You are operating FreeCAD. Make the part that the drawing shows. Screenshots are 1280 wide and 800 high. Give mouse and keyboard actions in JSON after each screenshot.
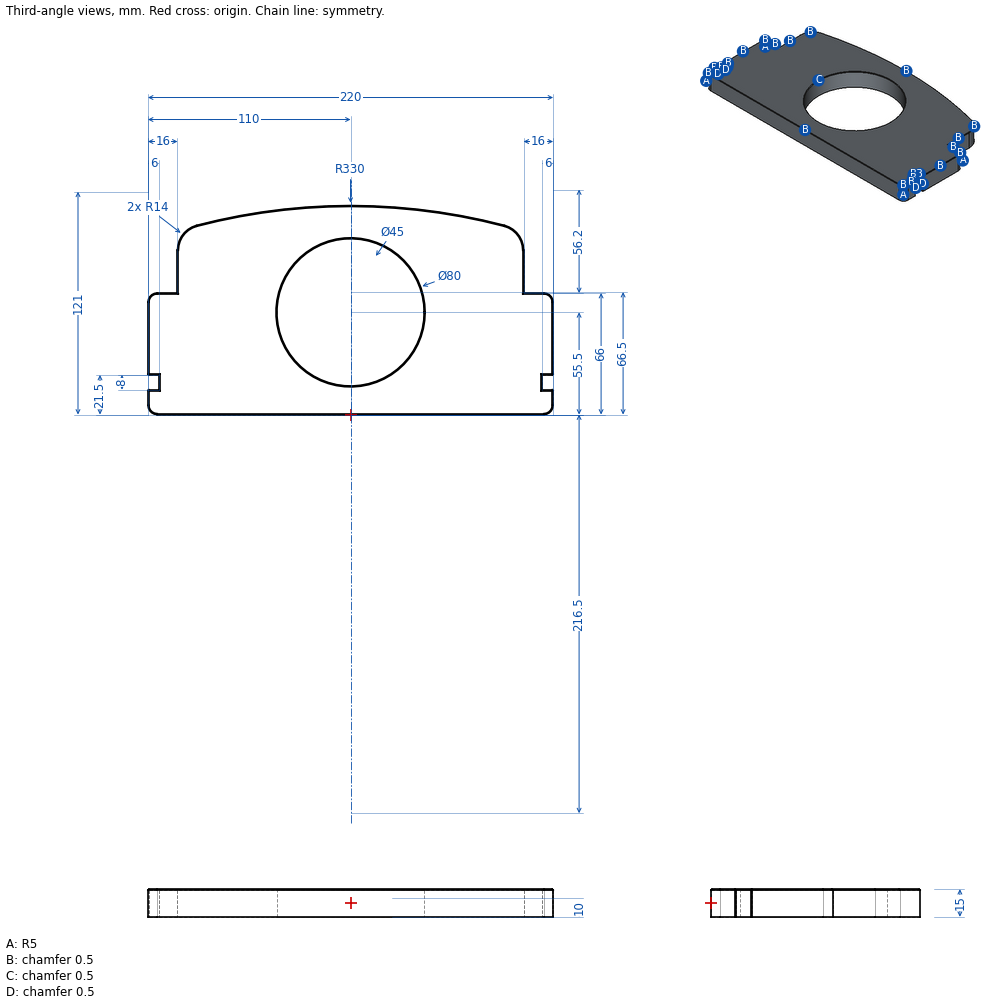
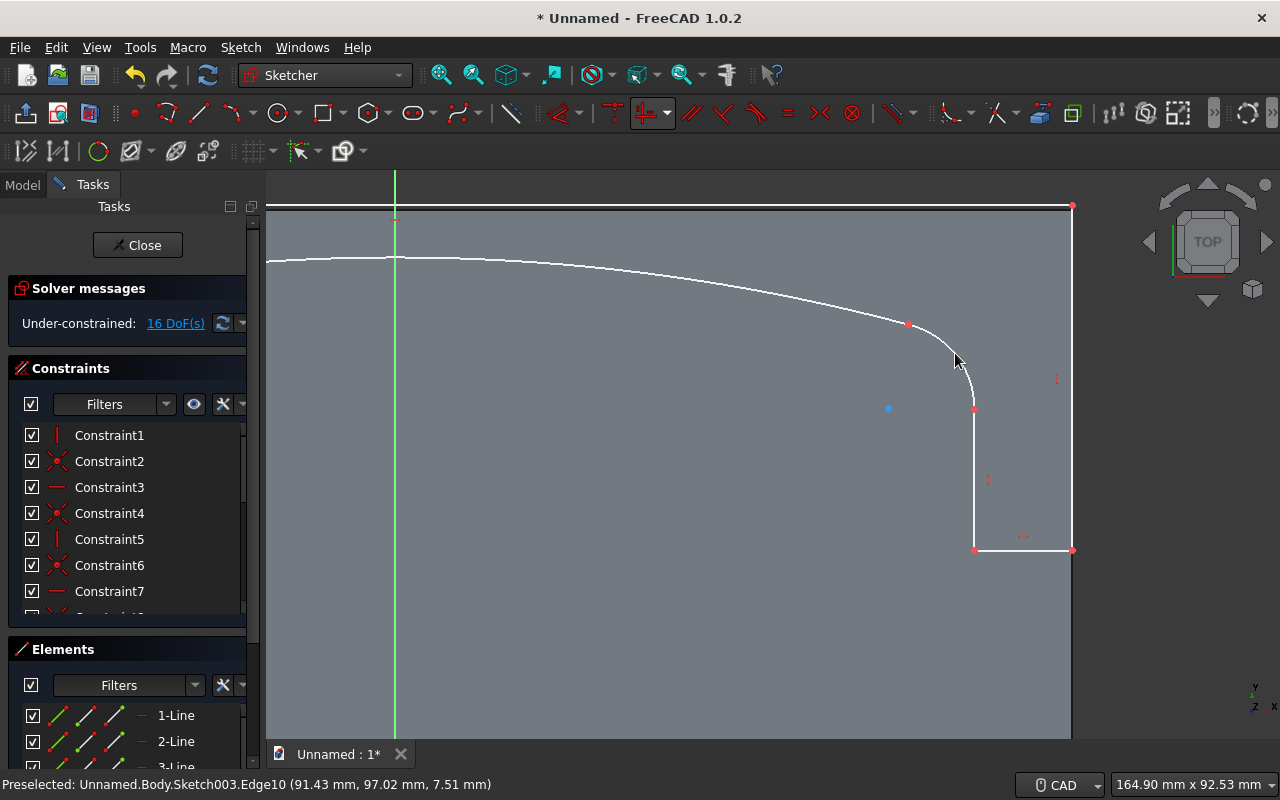
{"action": "left_click", "coordinate": [974, 452]}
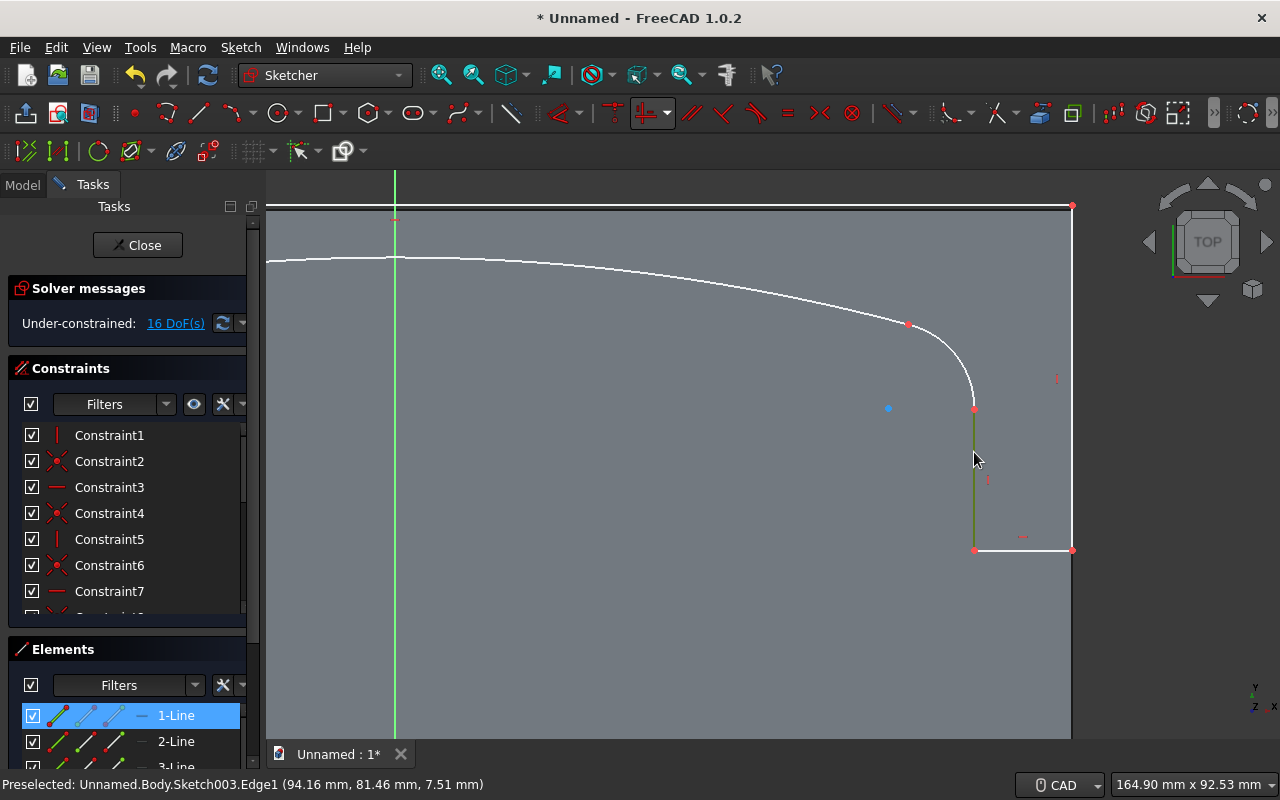
{"action": "left_click", "coordinate": [968, 375]}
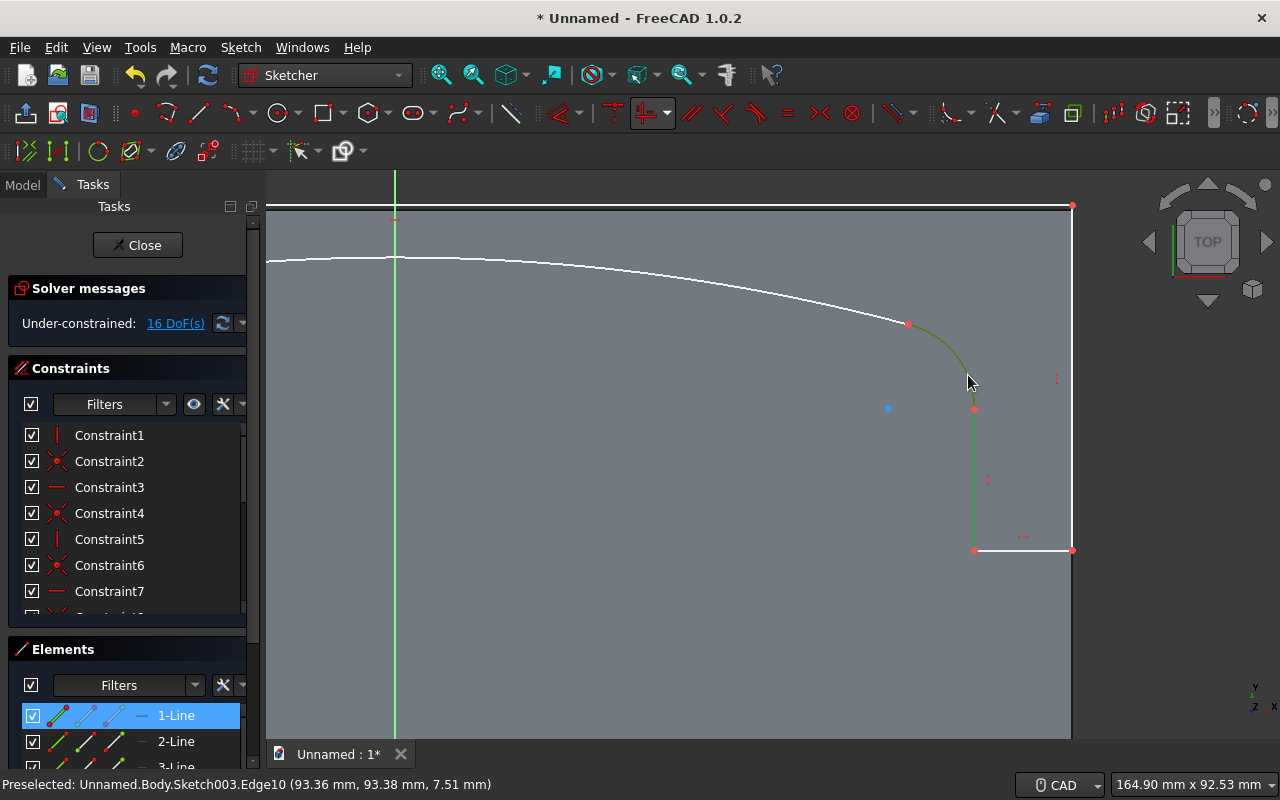
{"action": "left_click", "coordinate": [756, 114]}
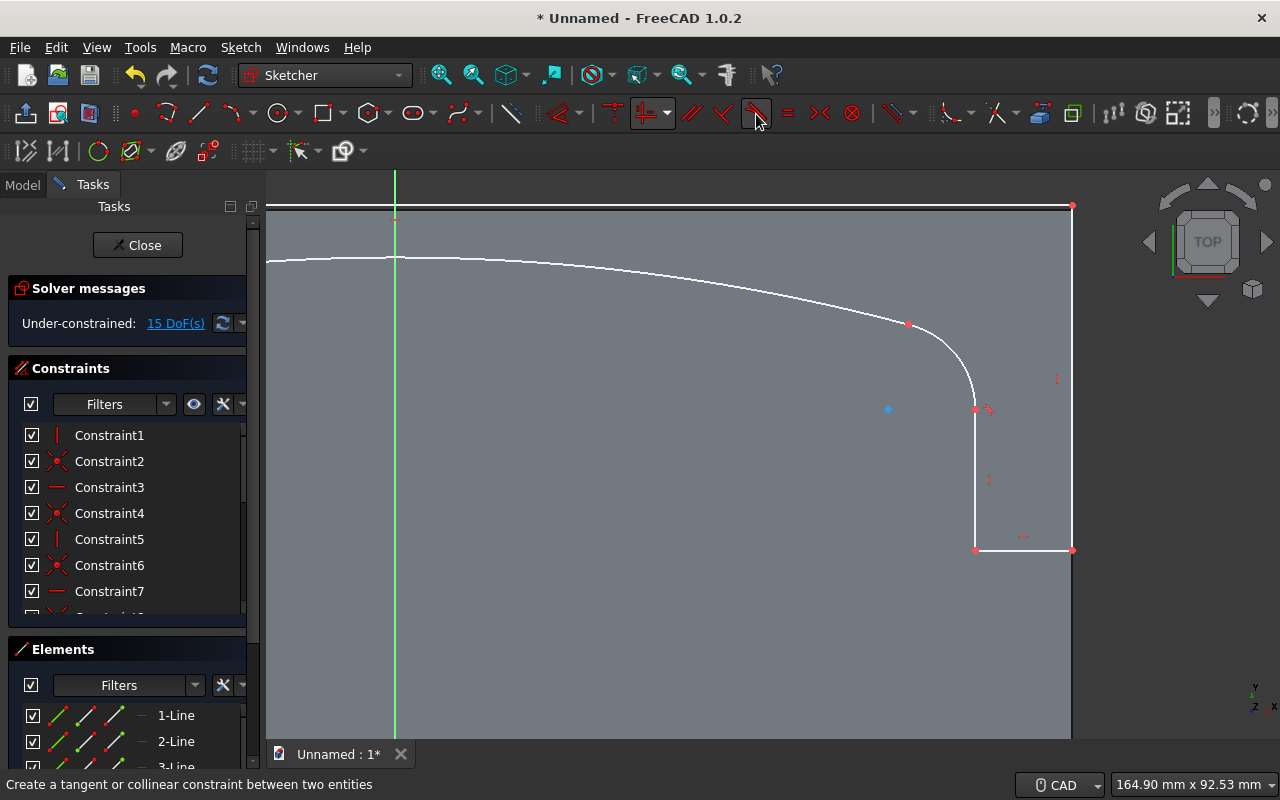
{"action": "scroll", "coordinate": [957, 354], "scroll_direction": "down", "scroll_amount": 4}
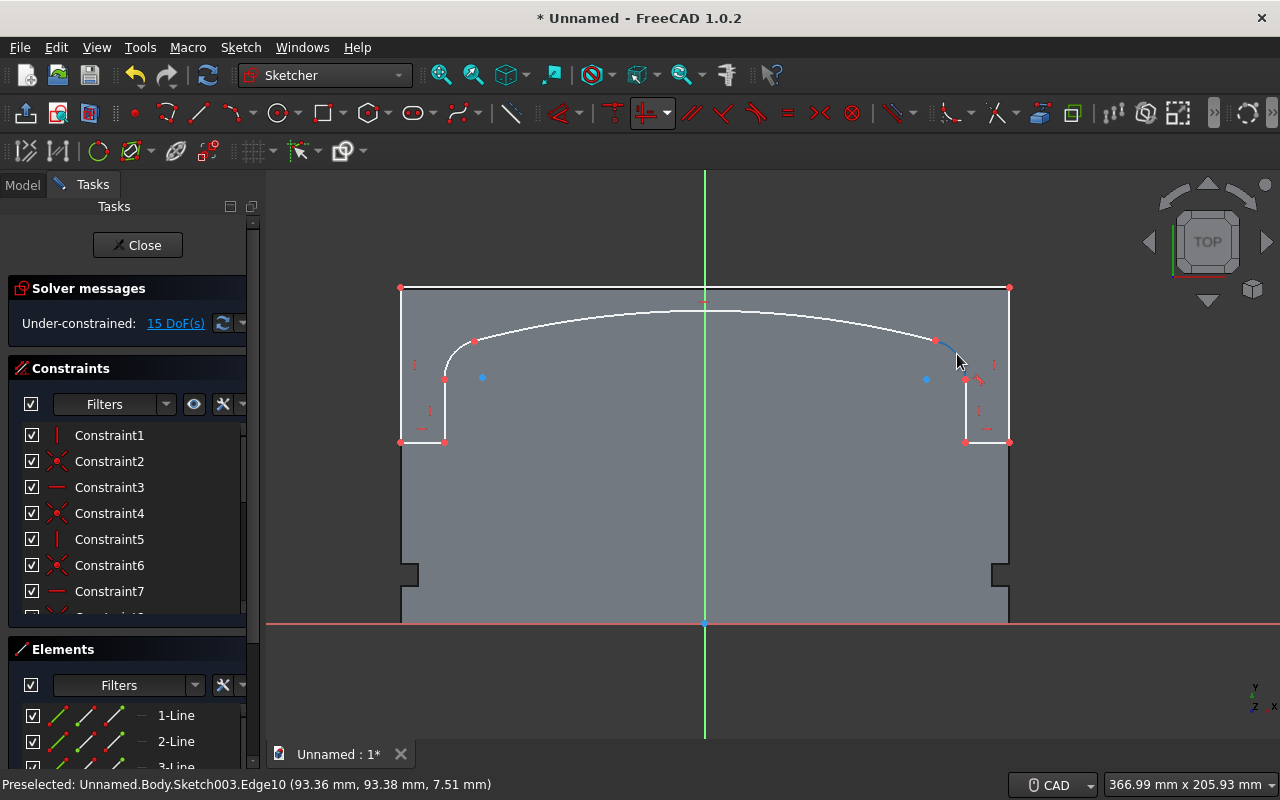
{"action": "left_click", "coordinate": [445, 423]}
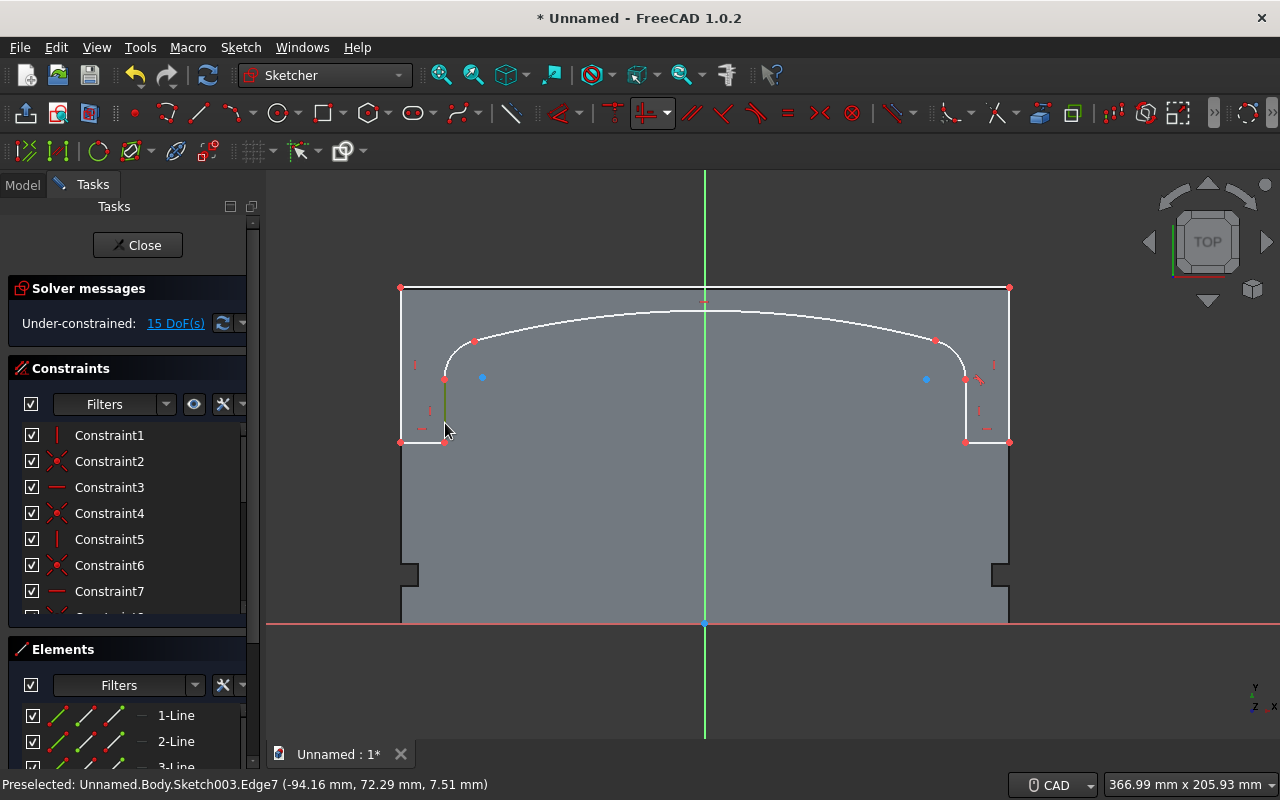
{"action": "left_click", "coordinate": [460, 348]}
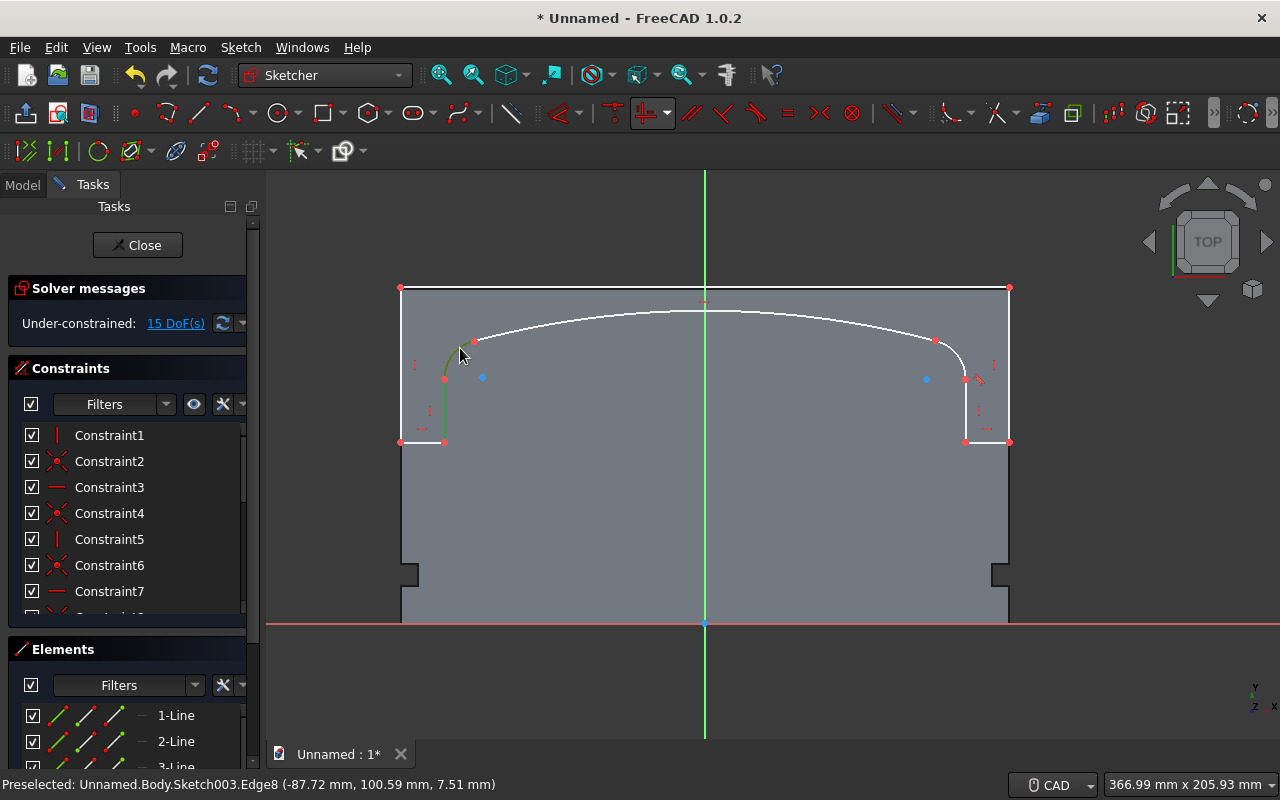
{"action": "left_click", "coordinate": [756, 114]}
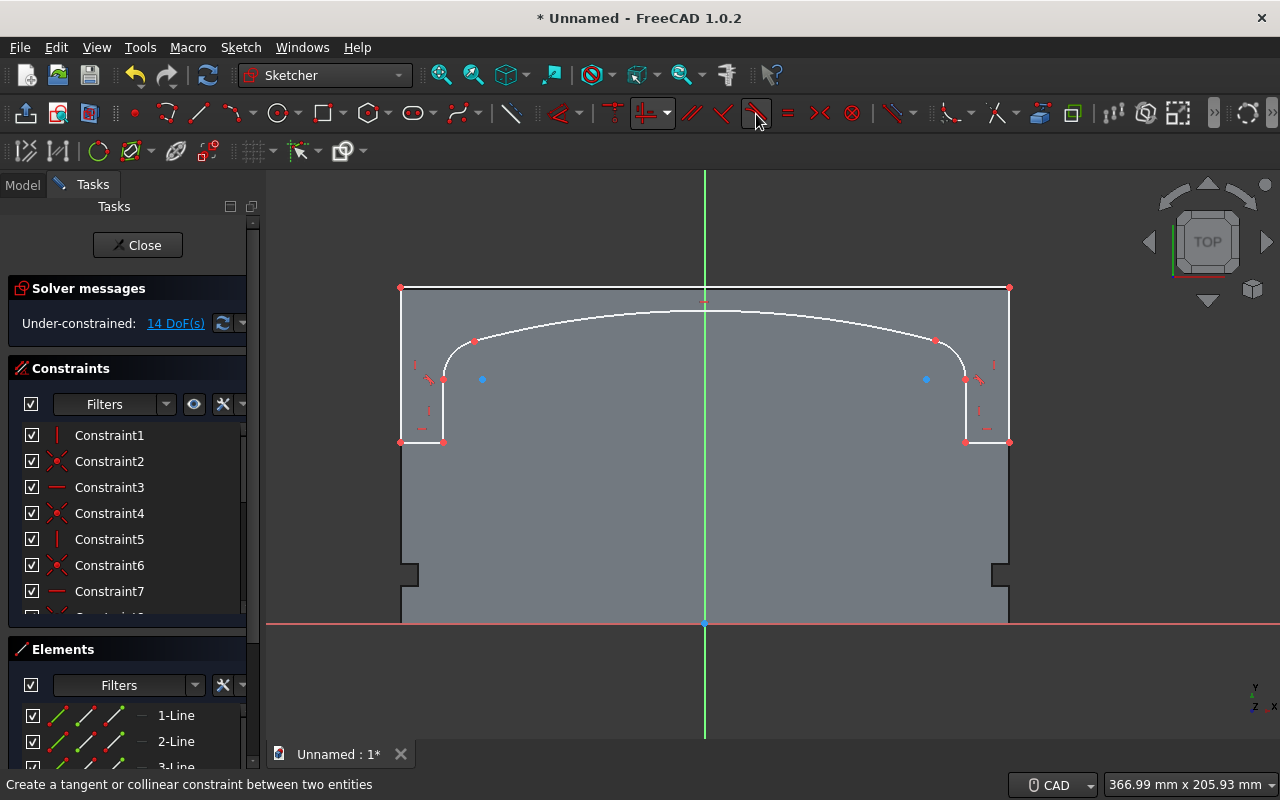
{"action": "left_click", "coordinate": [460, 347]}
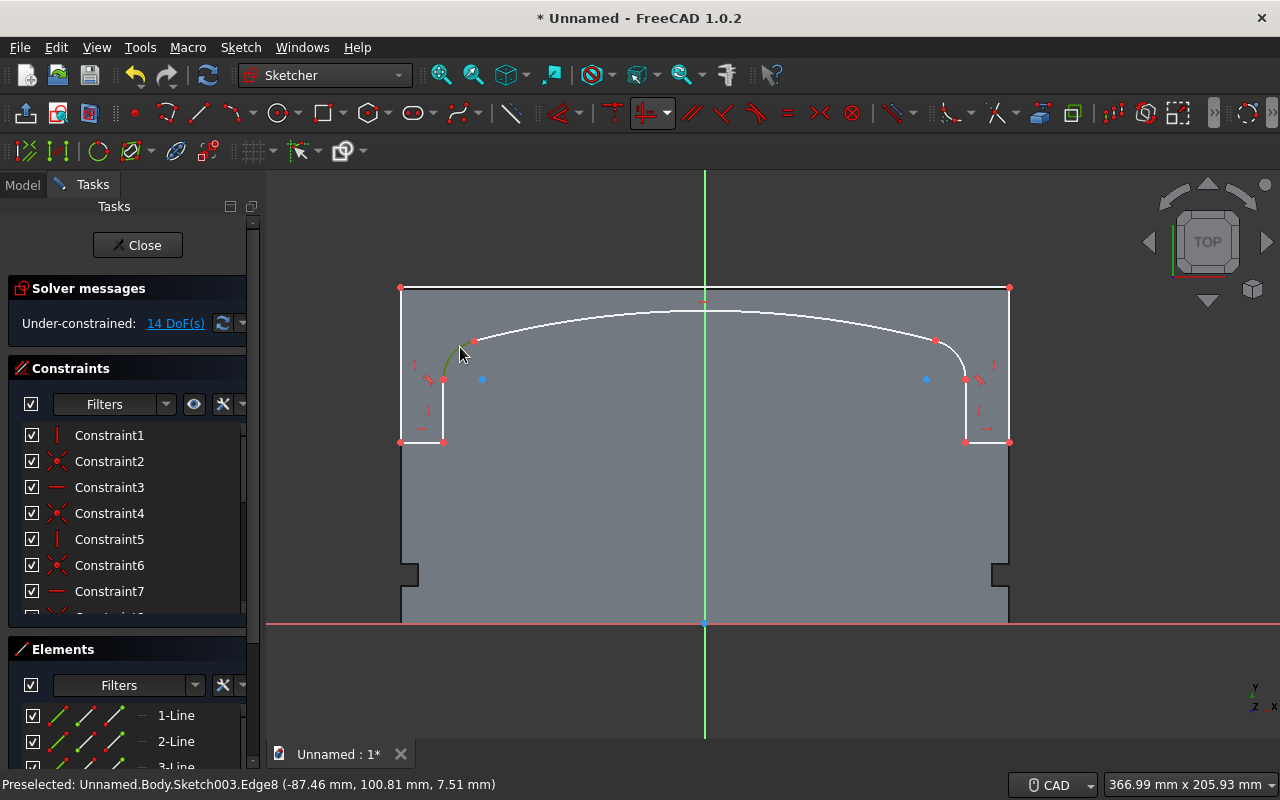
{"action": "left_click", "coordinate": [798, 316]}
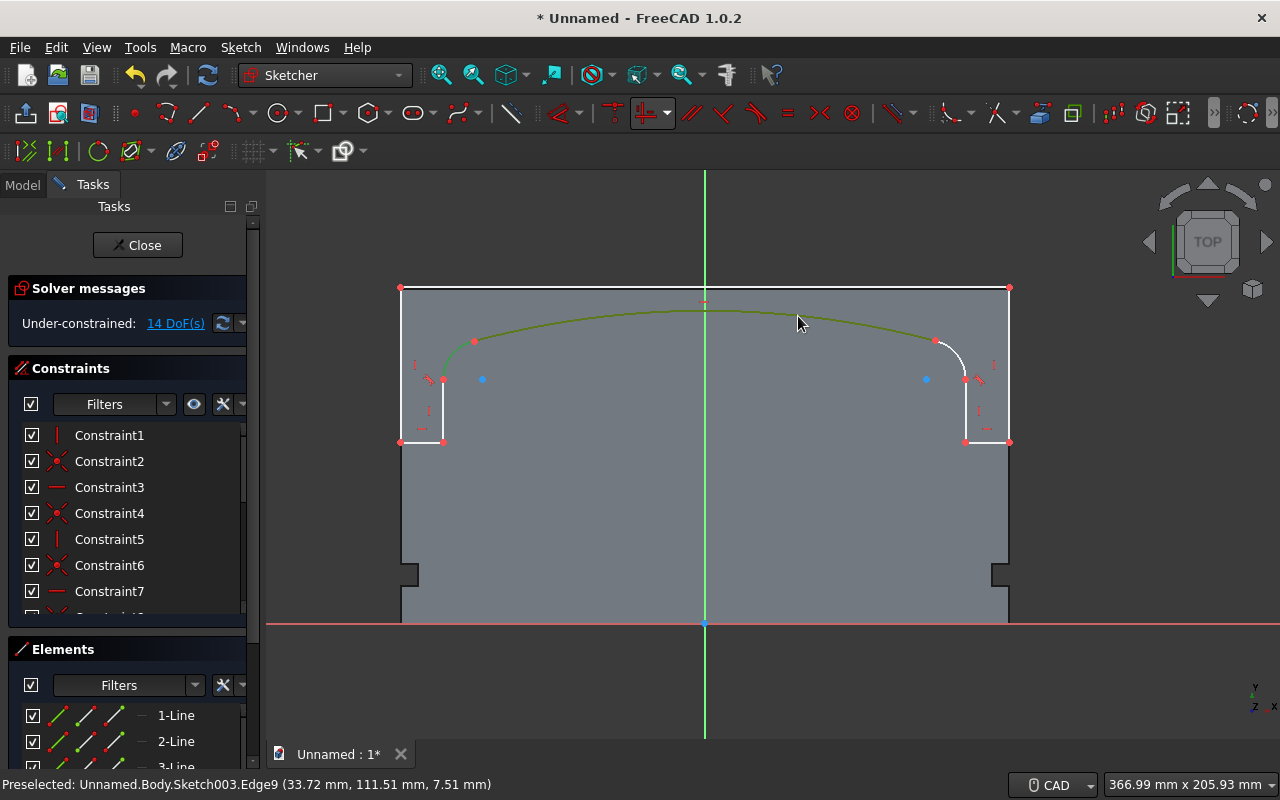
{"action": "left_click", "coordinate": [756, 114]}